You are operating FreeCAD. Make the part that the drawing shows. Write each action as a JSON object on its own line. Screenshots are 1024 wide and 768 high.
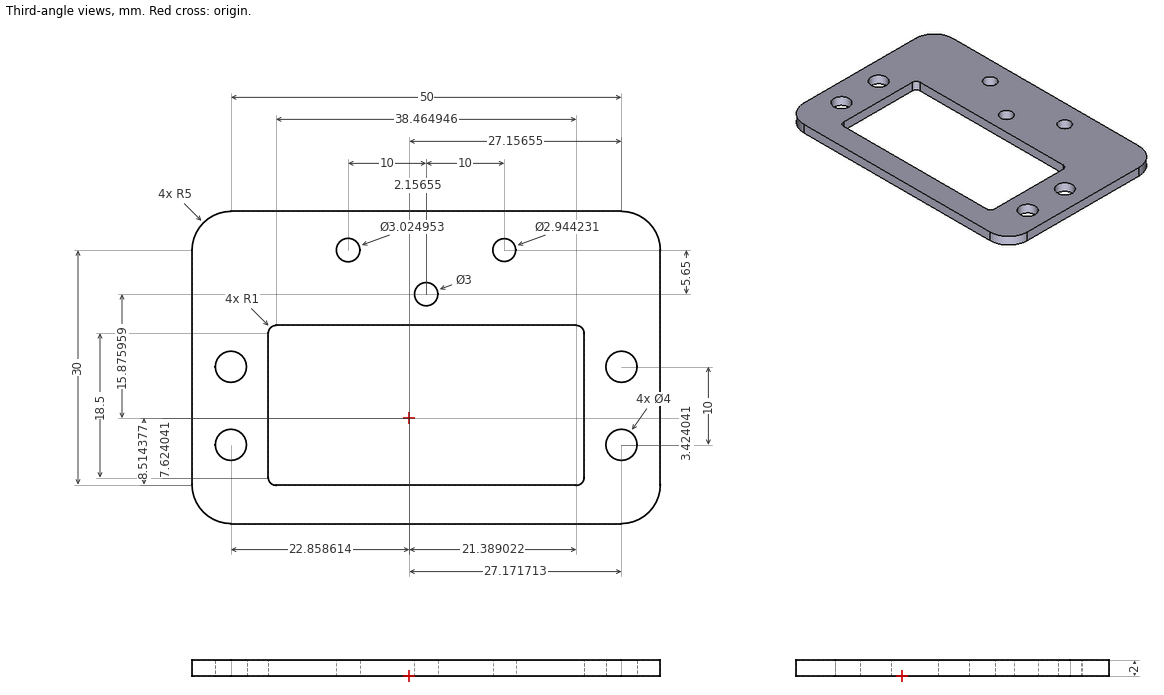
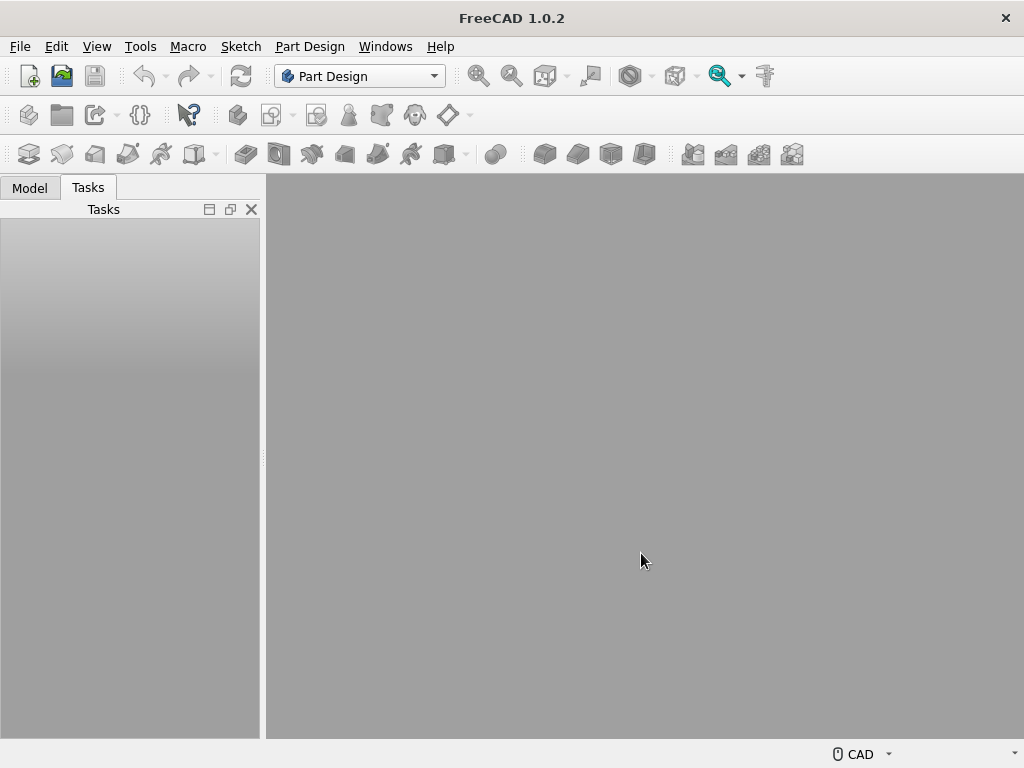
{"action": "left_click", "coordinate": [29, 76]}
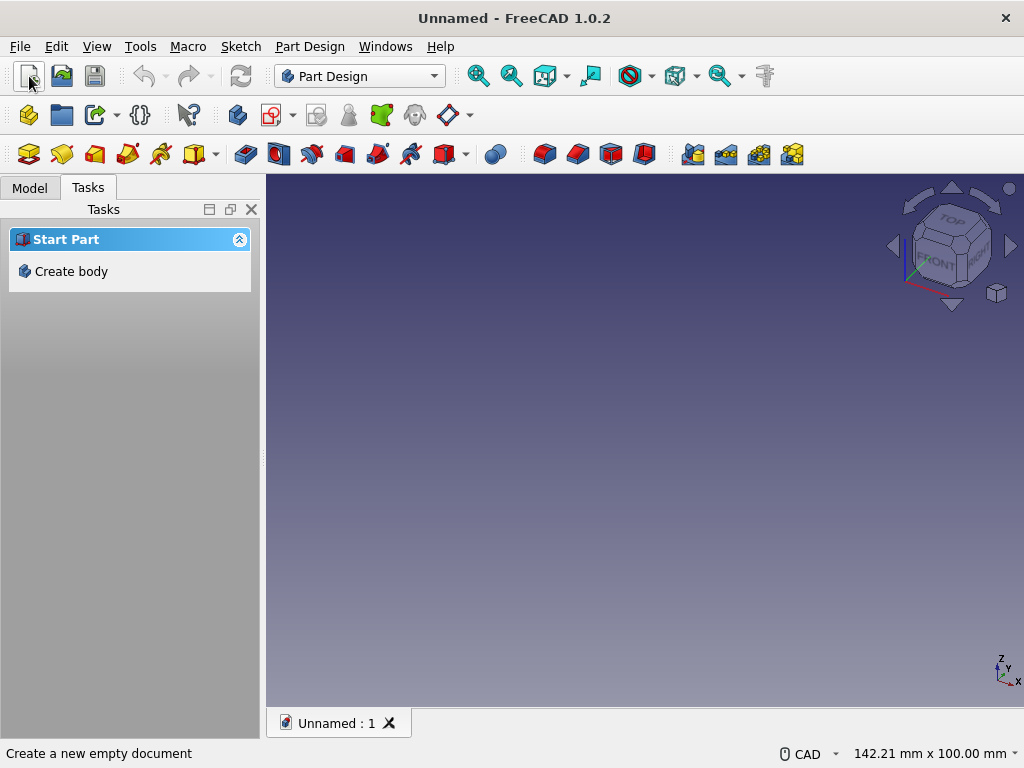
{"action": "left_click", "coordinate": [270, 116]}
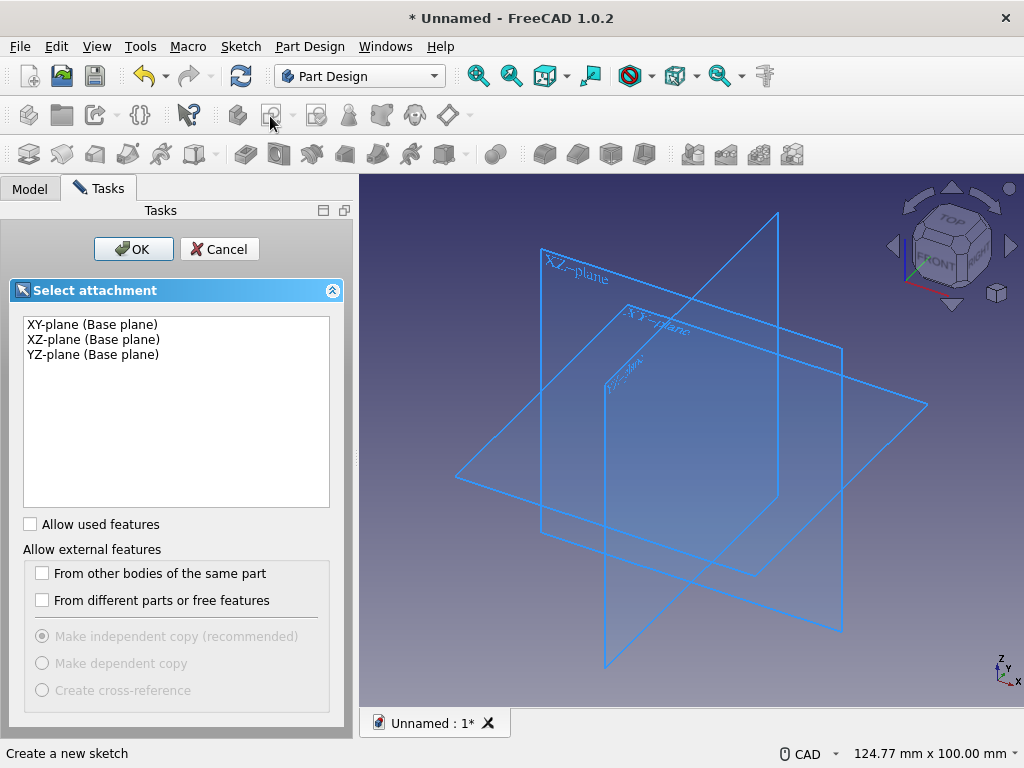
{"action": "left_click", "coordinate": [84, 324]}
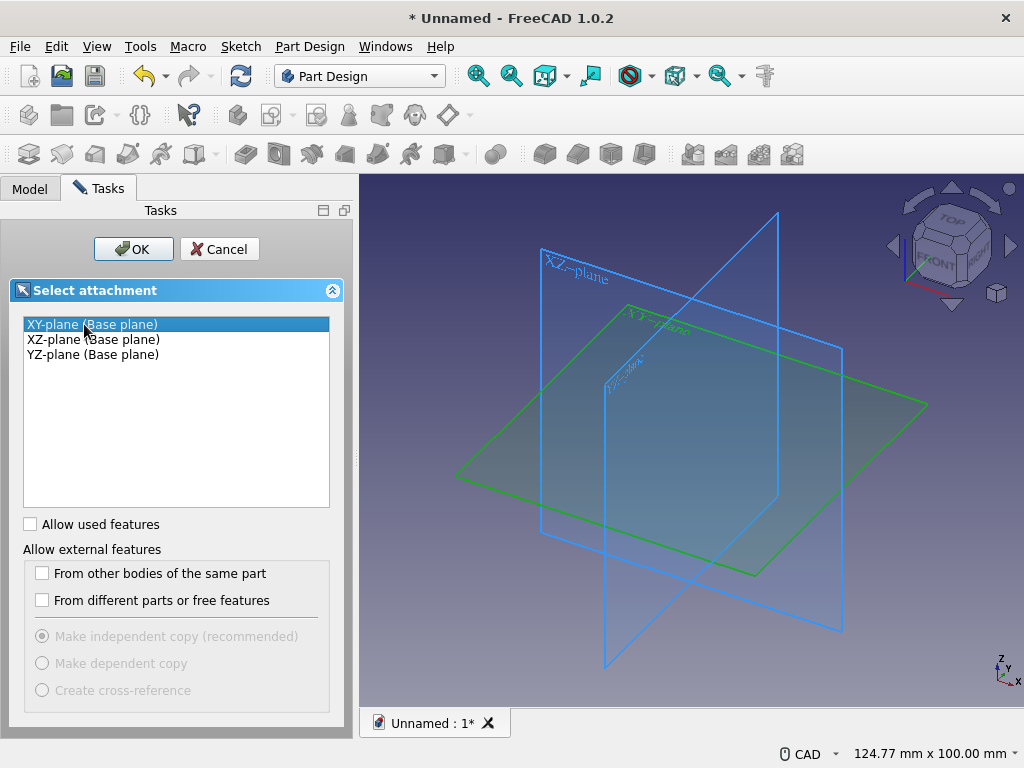
{"action": "left_click", "coordinate": [134, 249]}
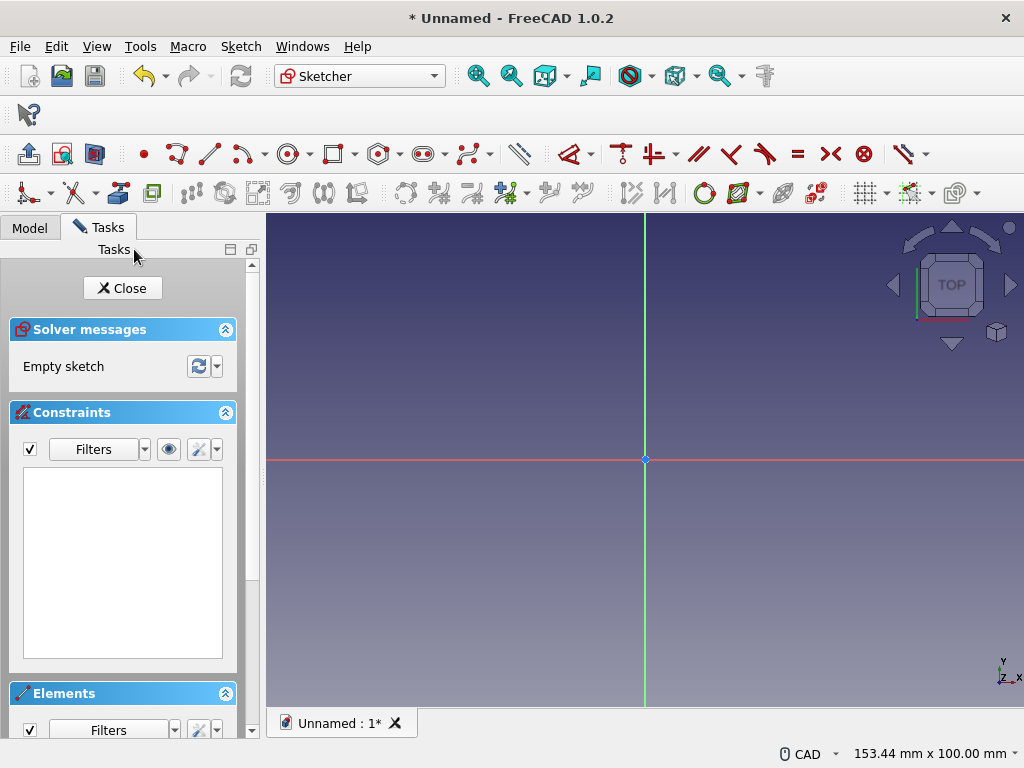
{"action": "left_click", "coordinate": [210, 154]}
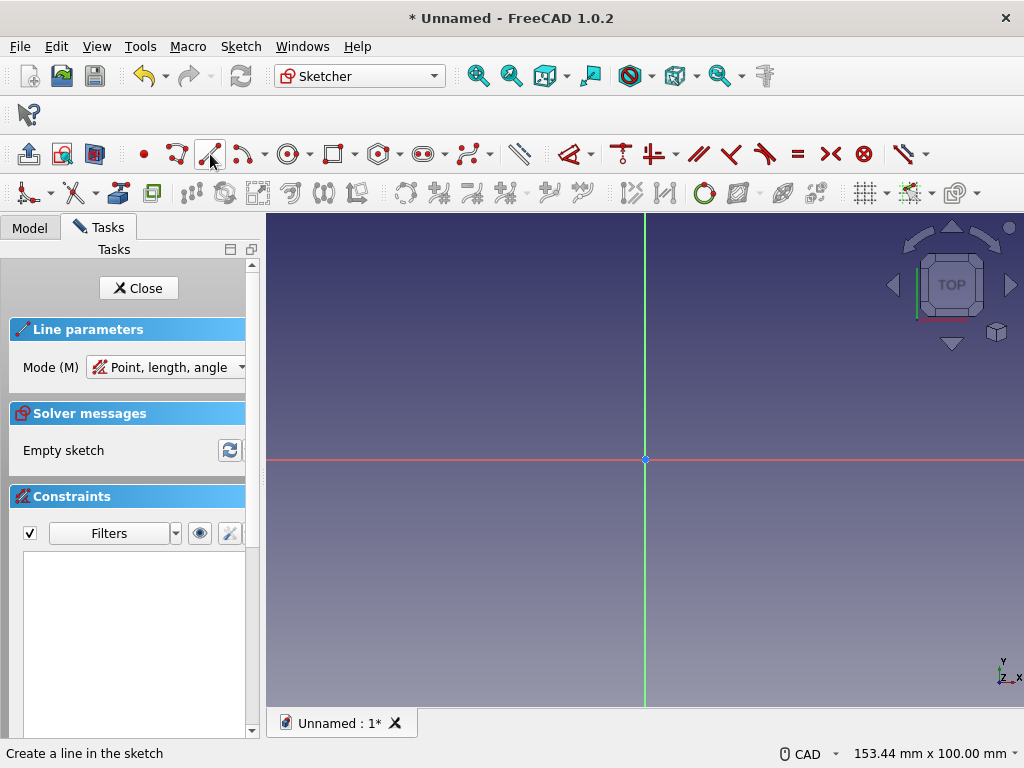
{"action": "left_click", "coordinate": [779, 329]}
{"action": "left_click", "coordinate": [532, 329]}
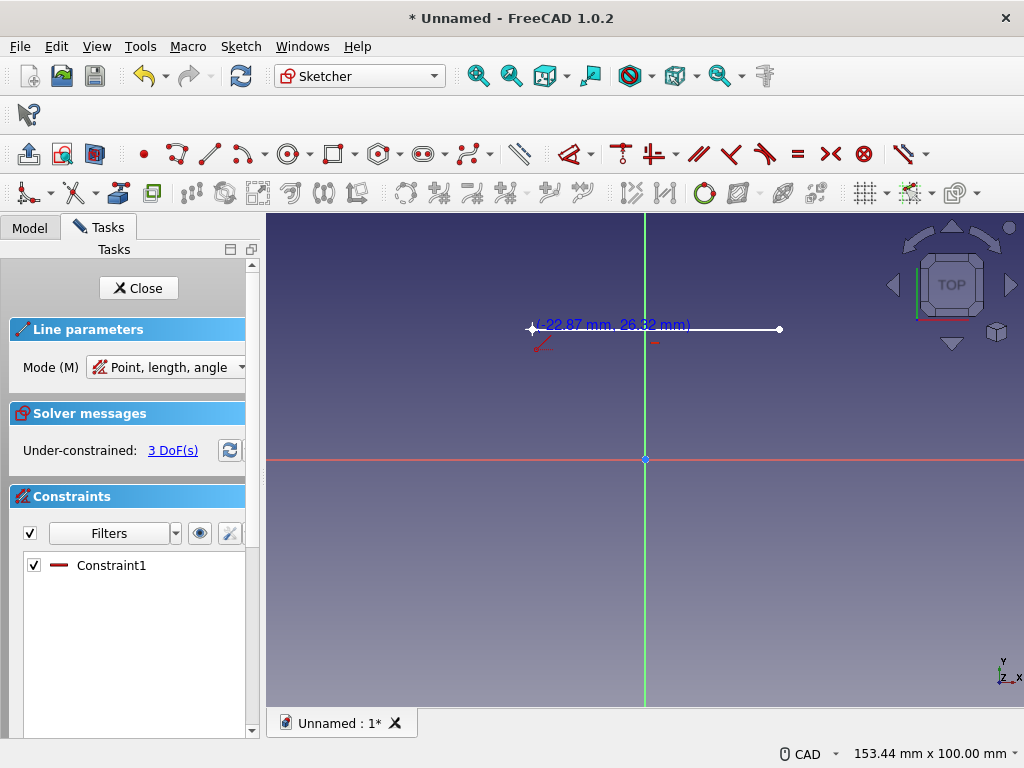
{"action": "left_click", "coordinate": [507, 354]}
{"action": "left_click", "coordinate": [507, 502]}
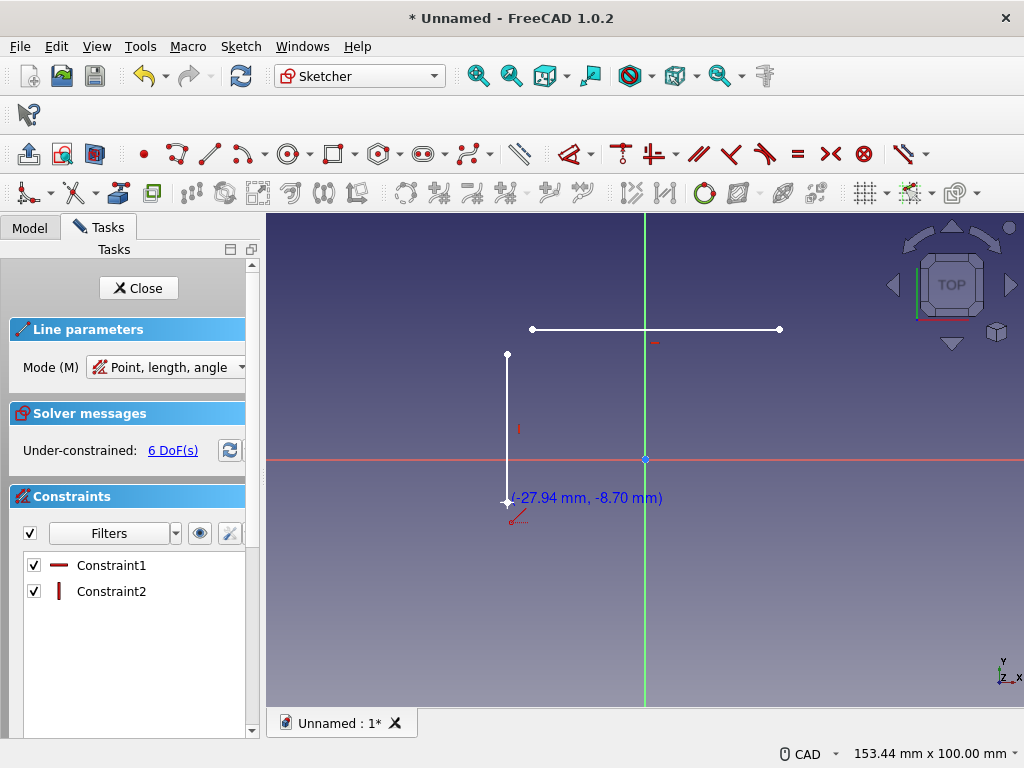
{"action": "left_click", "coordinate": [532, 527]}
{"action": "left_click", "coordinate": [779, 527]}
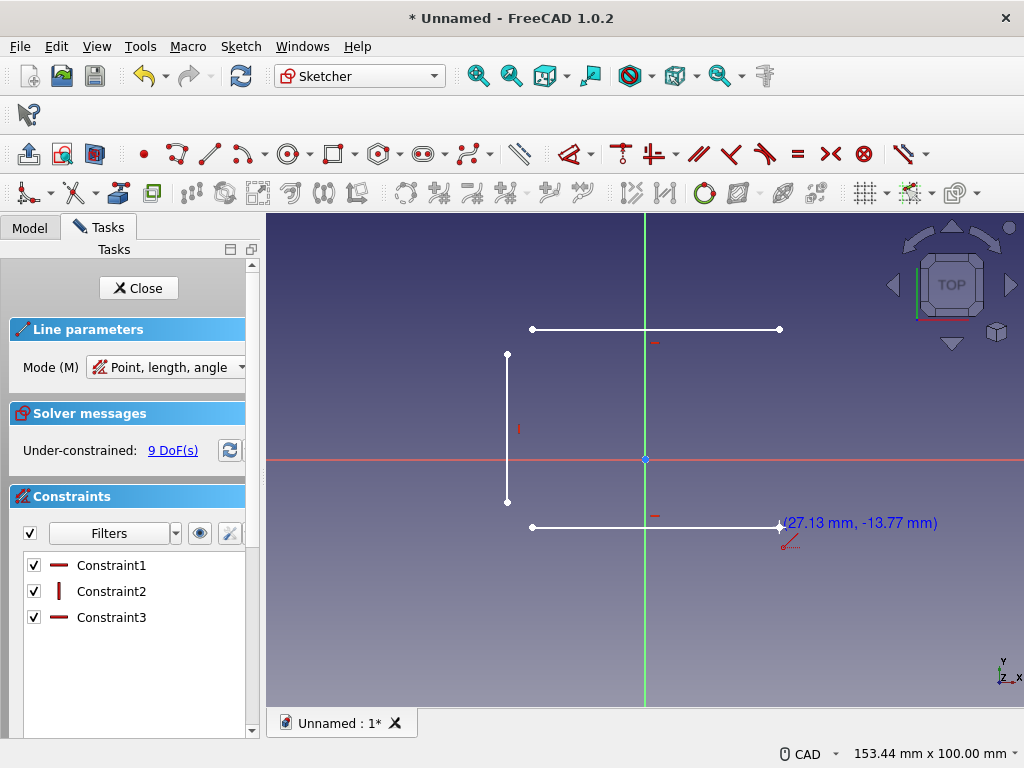
{"action": "left_click", "coordinate": [804, 502]}
{"action": "left_click", "coordinate": [804, 354]}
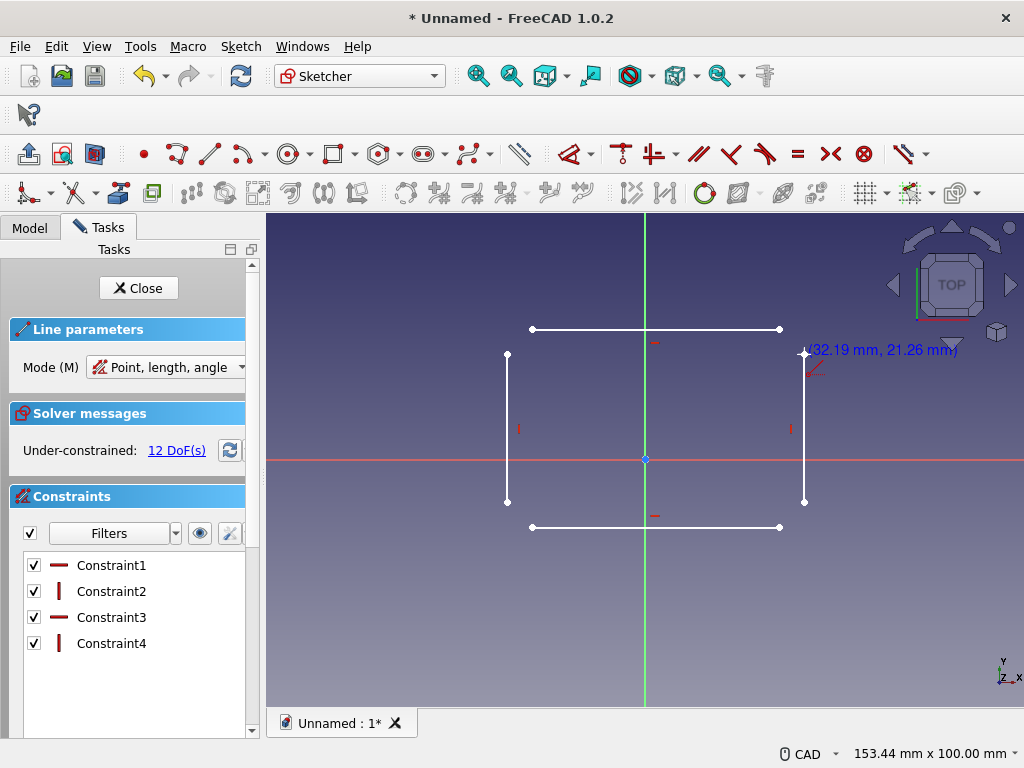
{"action": "left_click", "coordinate": [264, 154]}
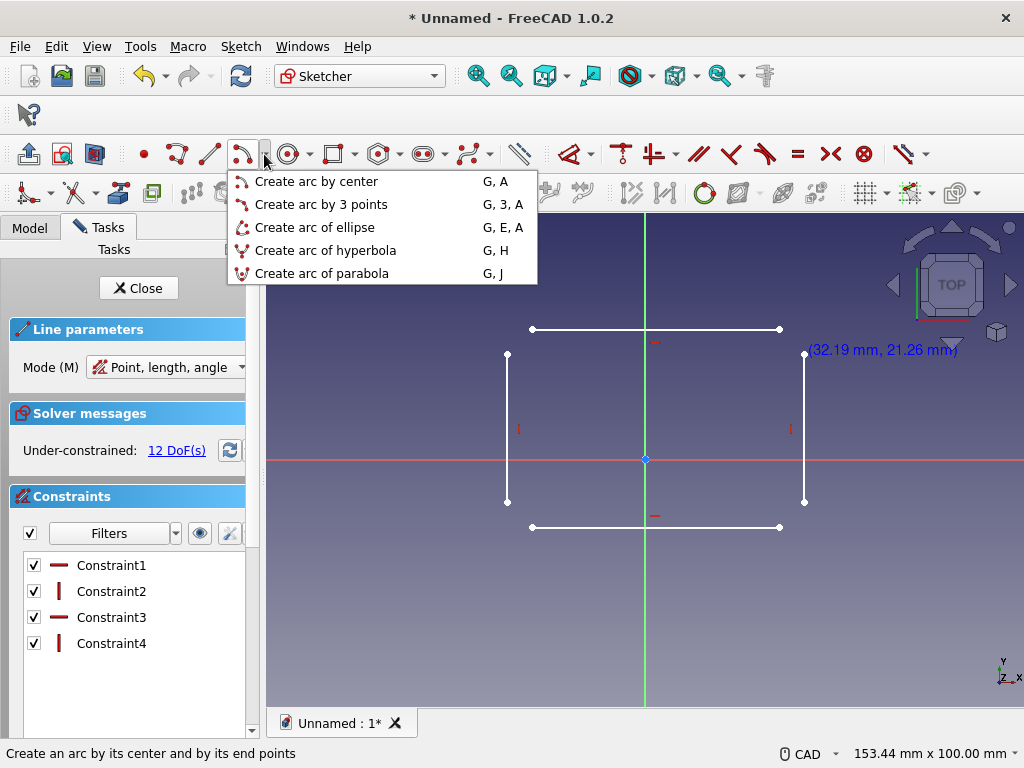
{"action": "left_click", "coordinate": [382, 204]}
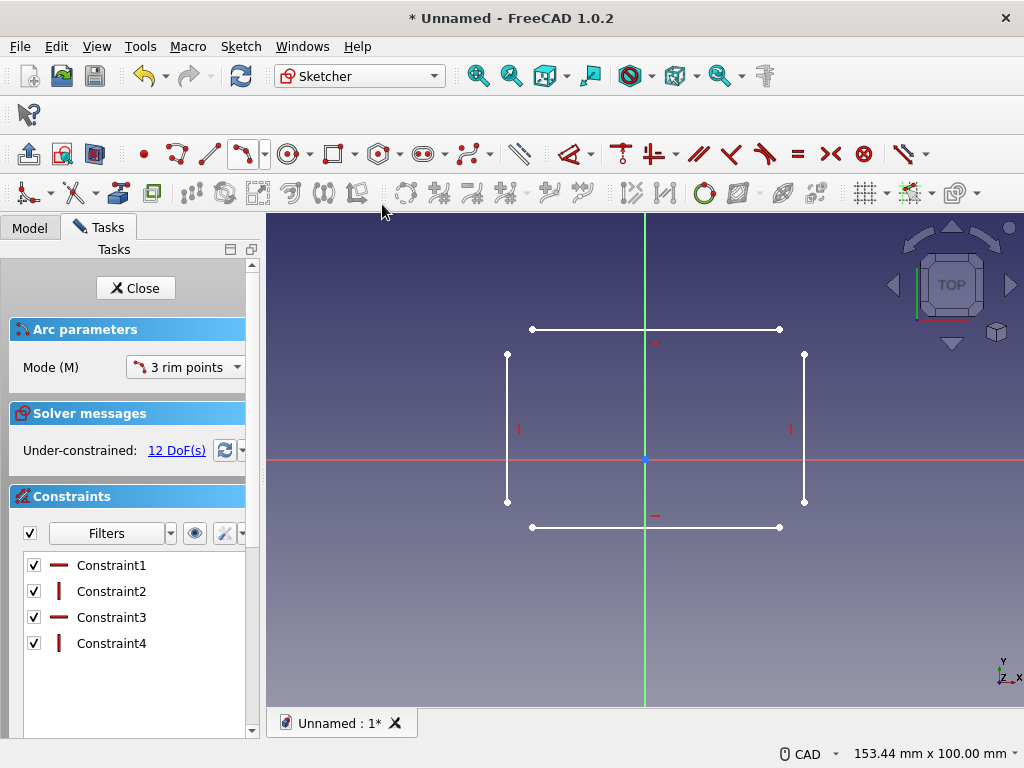
{"action": "left_click", "coordinate": [532, 330]}
{"action": "left_click", "coordinate": [507, 355]}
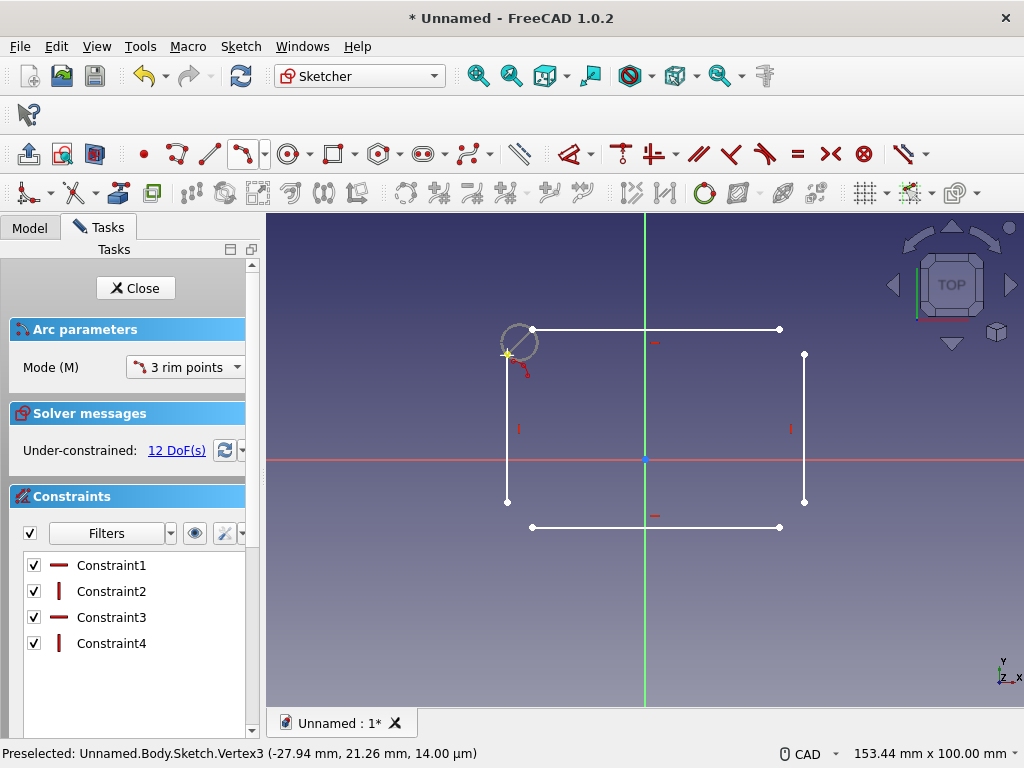
{"action": "scroll", "coordinate": [515, 336], "scroll_direction": "up", "scroll_amount": 4}